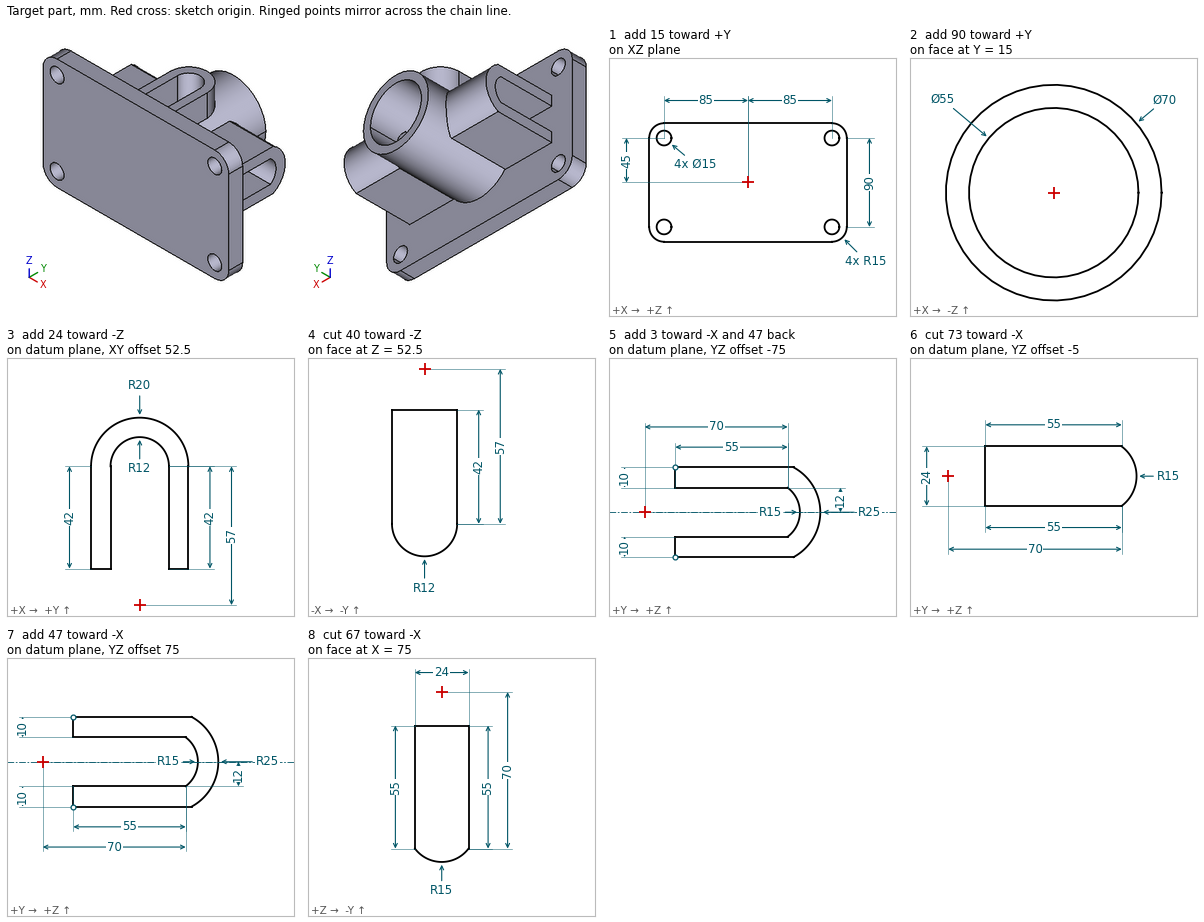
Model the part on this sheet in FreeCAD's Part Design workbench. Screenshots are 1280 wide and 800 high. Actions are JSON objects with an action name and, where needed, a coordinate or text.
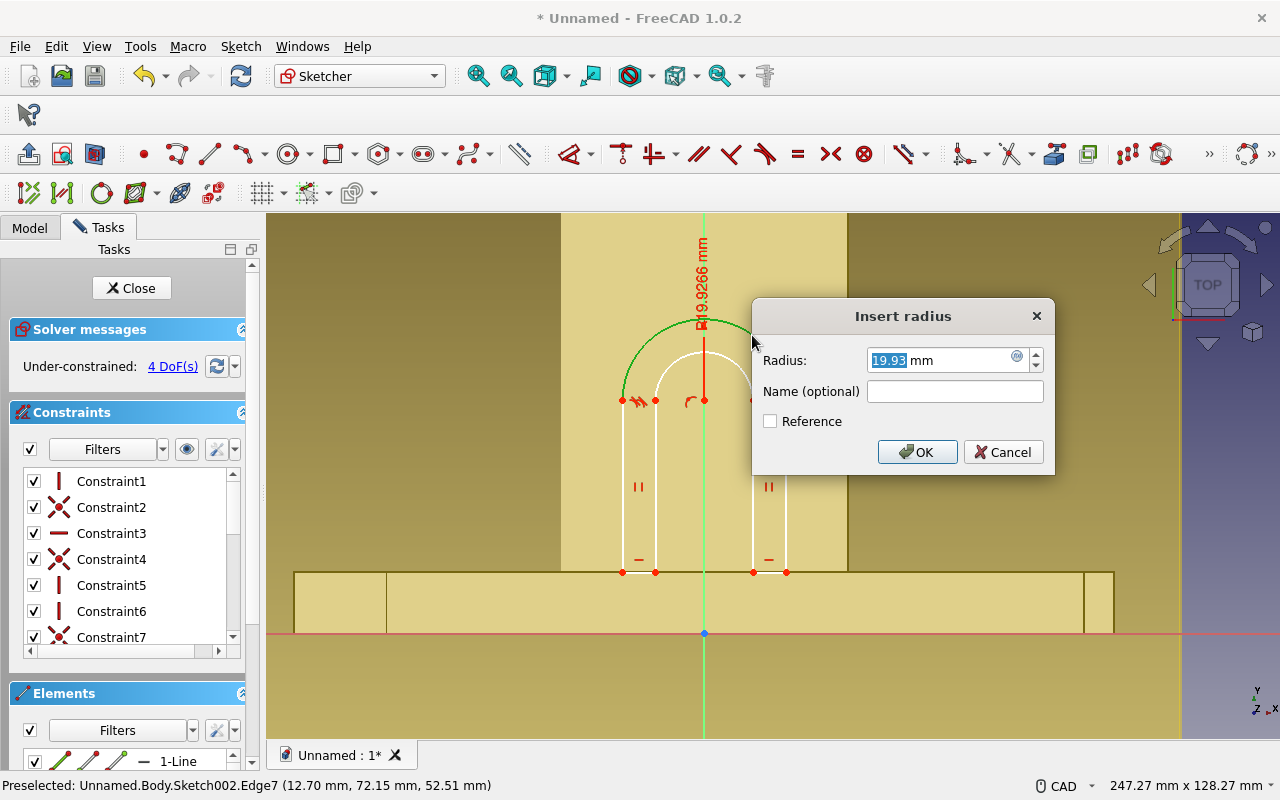
{"action": "type", "text": "20"}
{"action": "key", "text": "Return"}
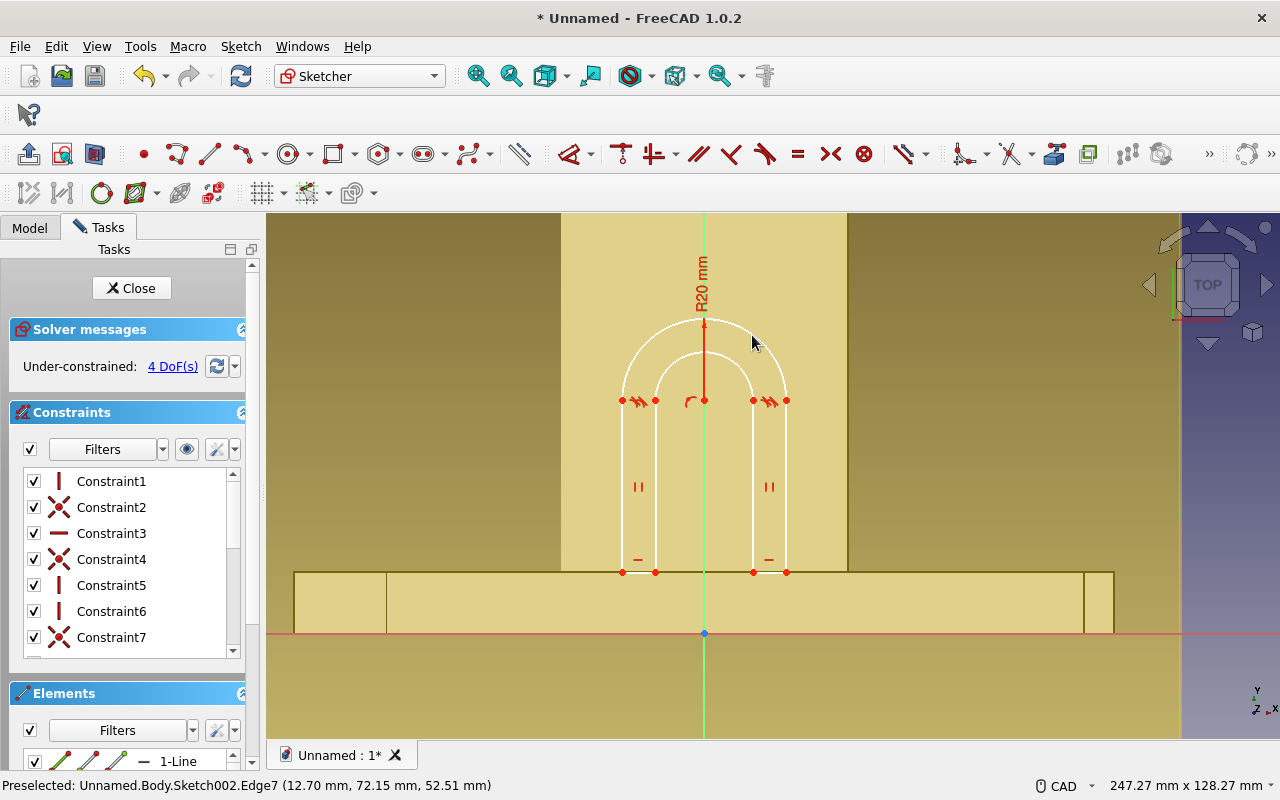
{"action": "left_click", "coordinate": [733, 362]}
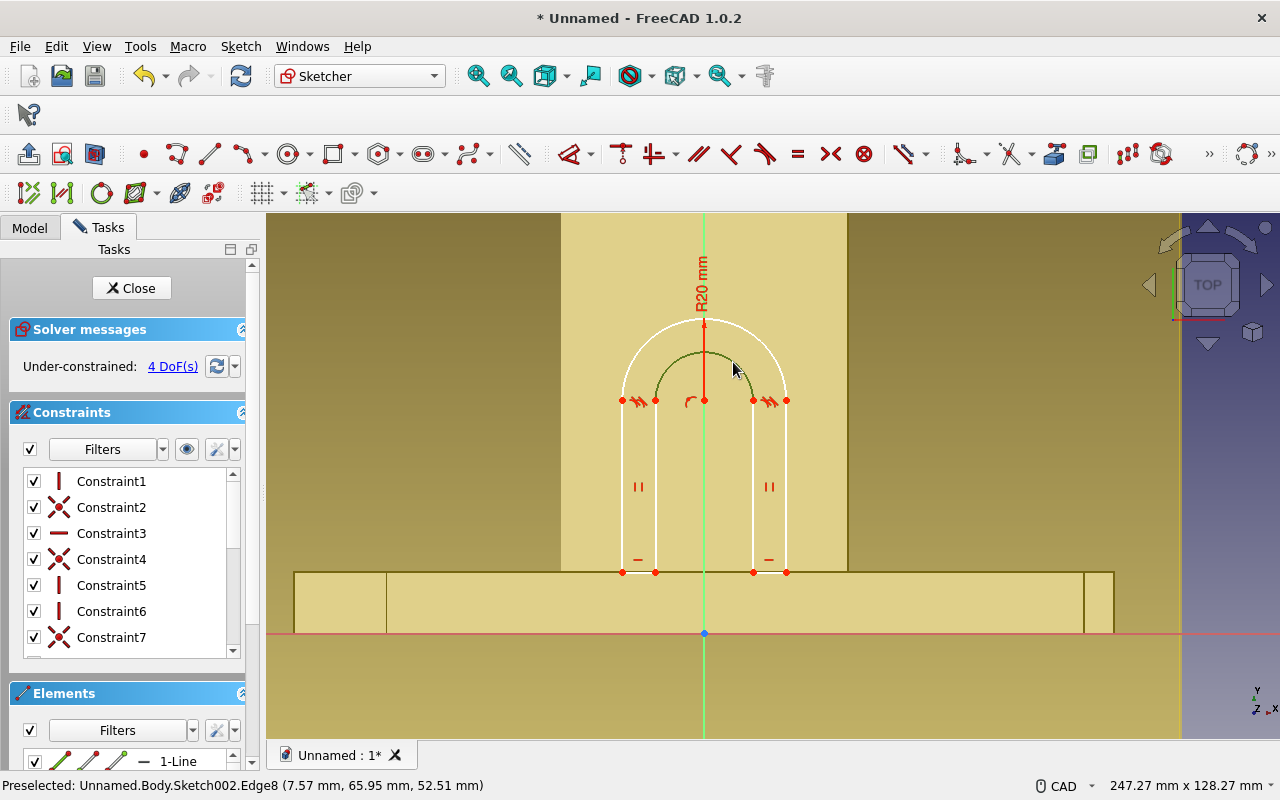
{"action": "key", "text": "k r"}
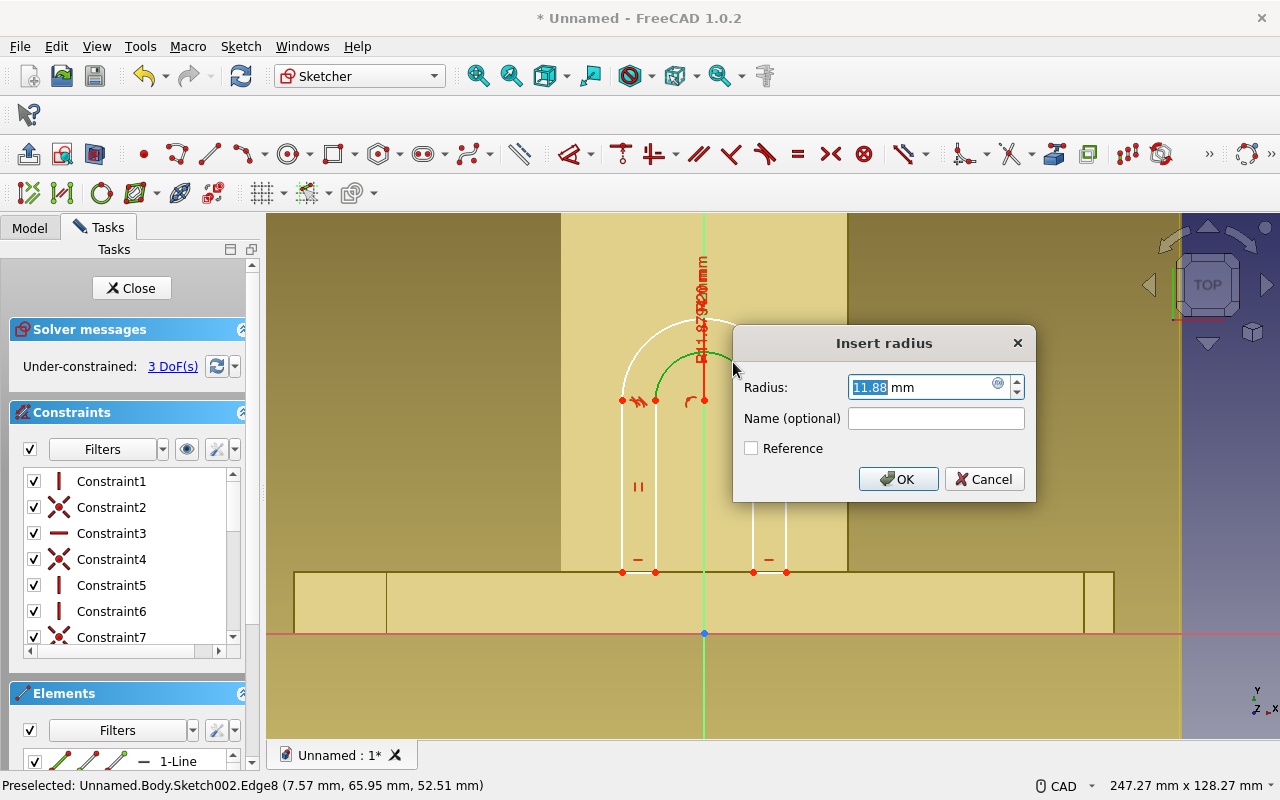
{"action": "type", "text": "12"}
{"action": "key", "text": "Return"}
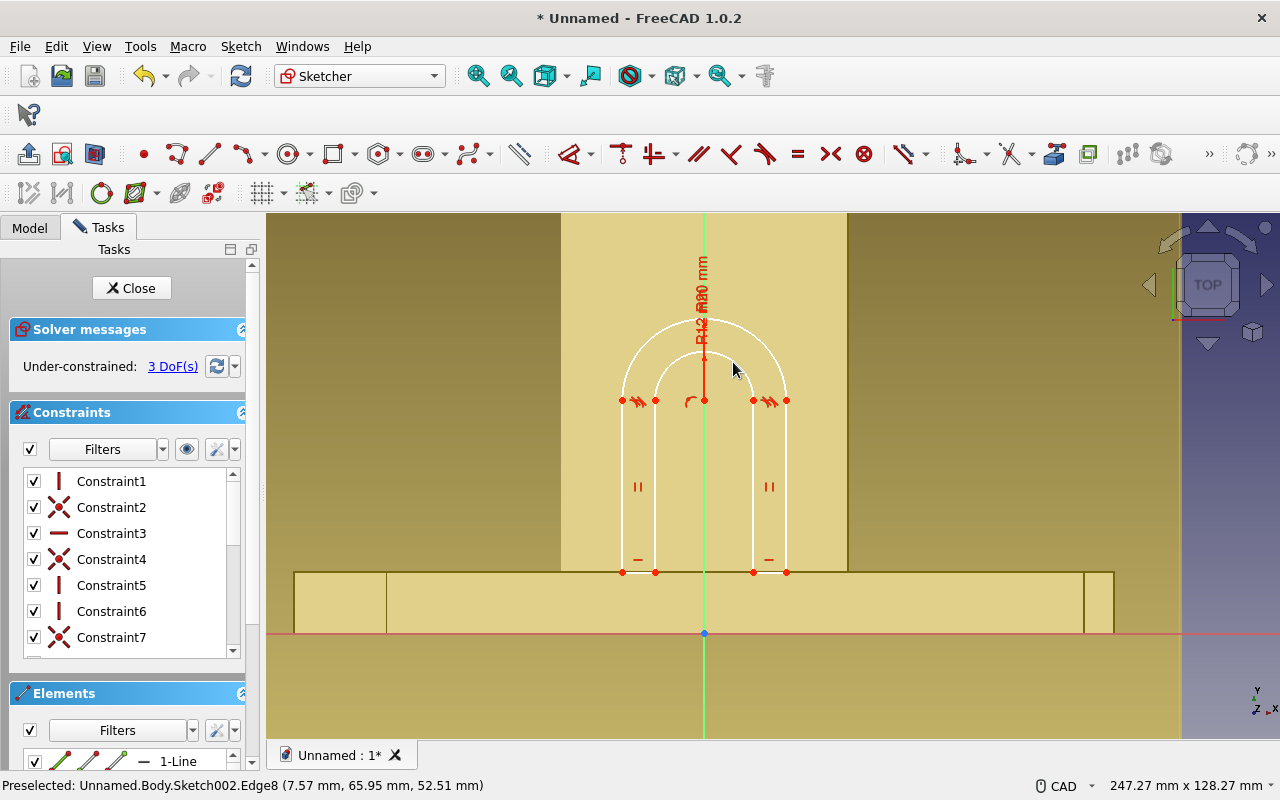
{"action": "left_click", "coordinate": [753, 453]}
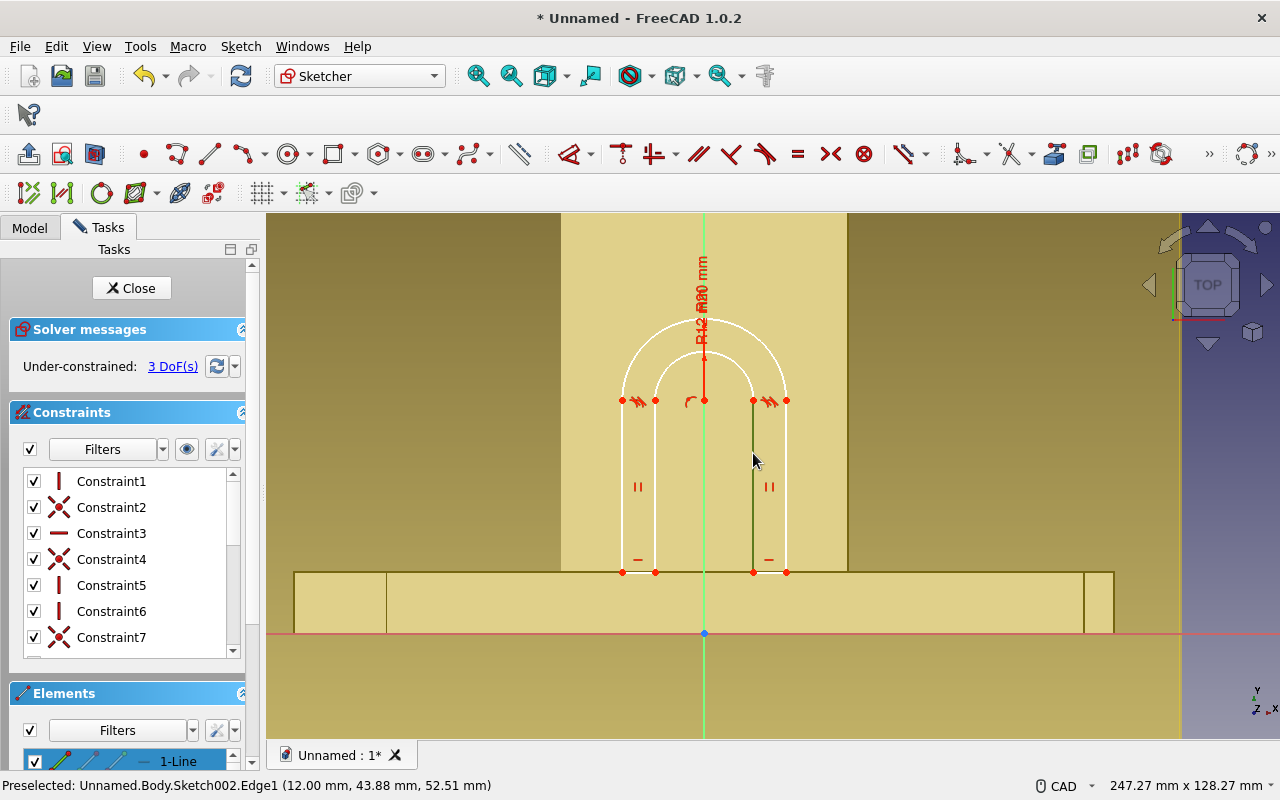
{"action": "key", "text": "i"}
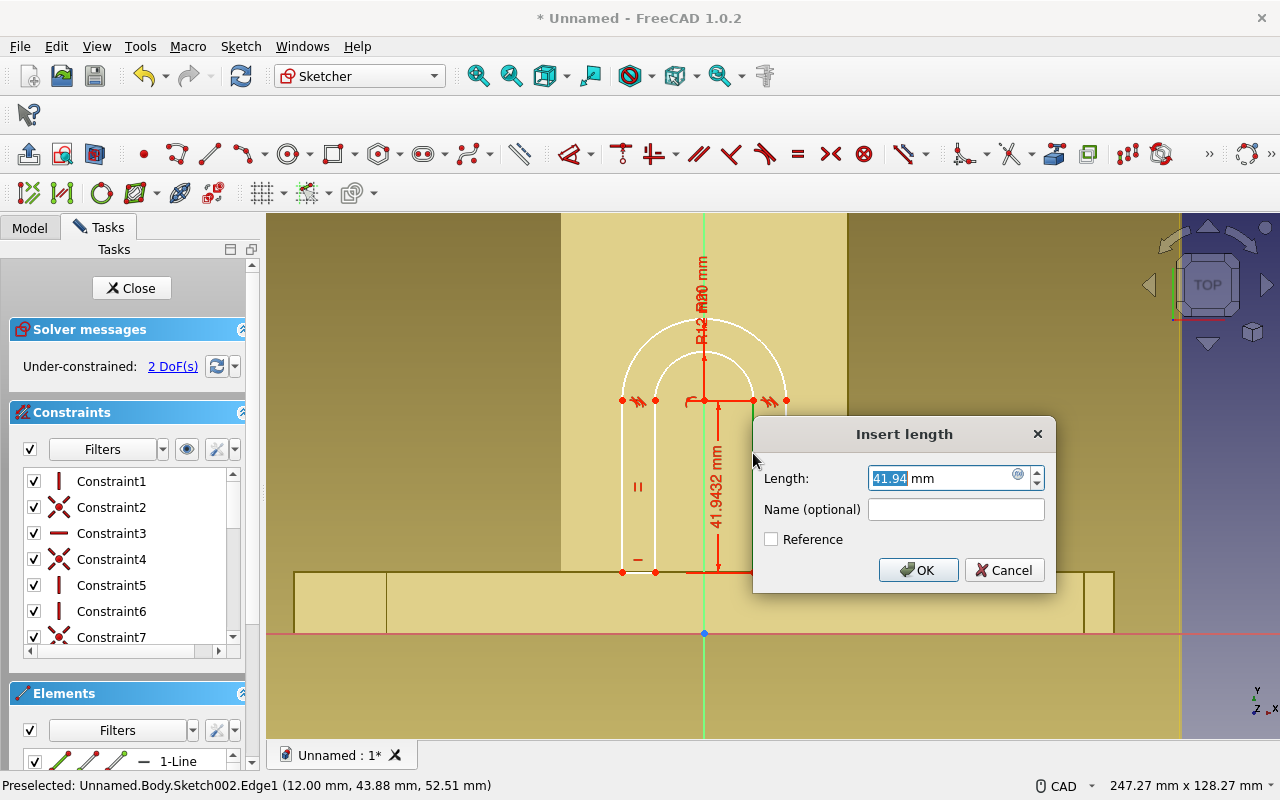
{"action": "type", "text": "42"}
{"action": "key", "text": "Return"}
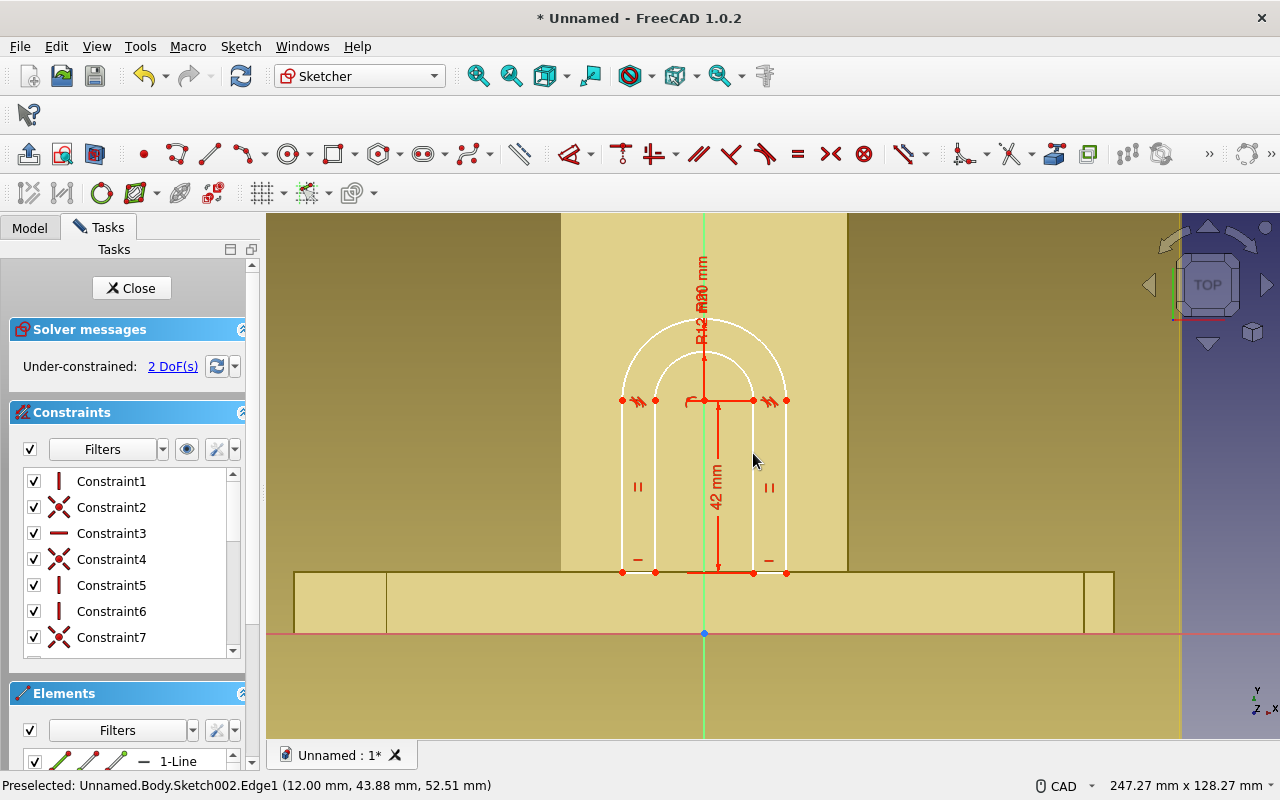
{"action": "left_click", "coordinate": [622, 453]}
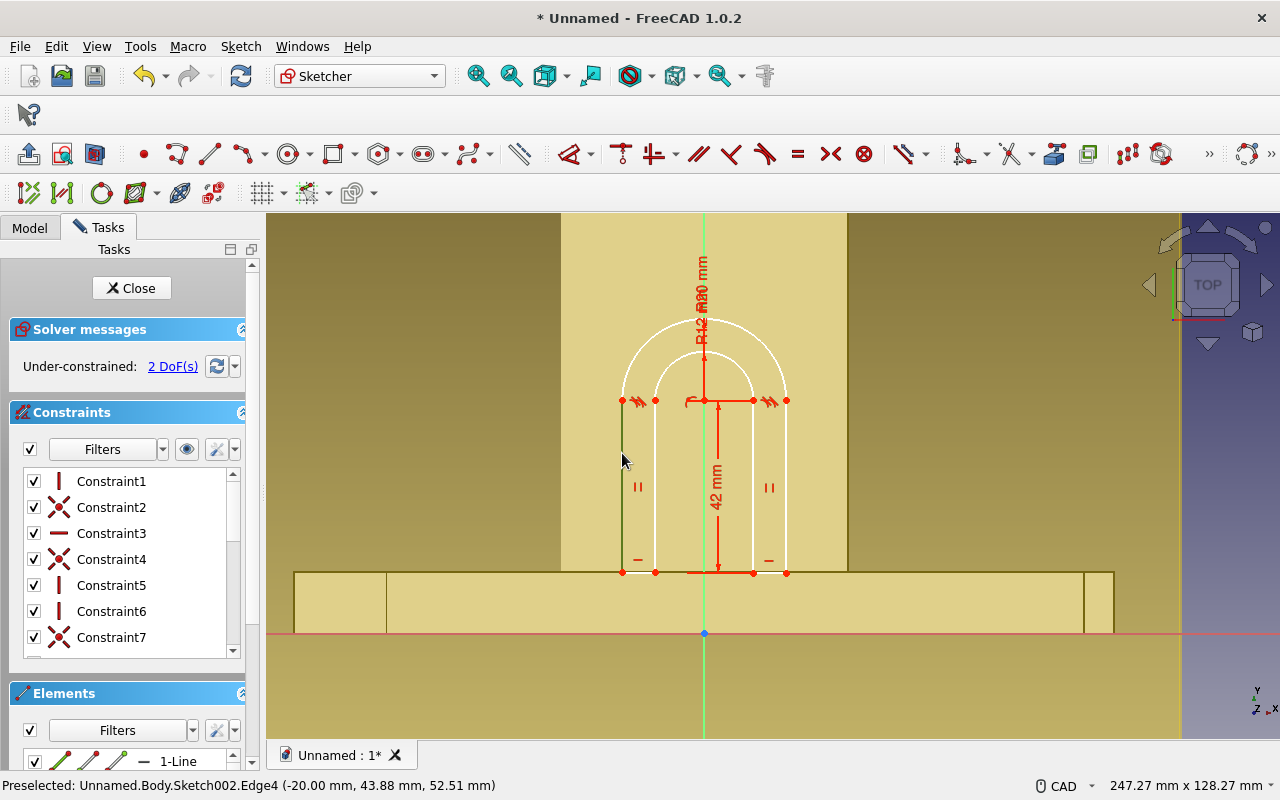
{"action": "key", "text": "i"}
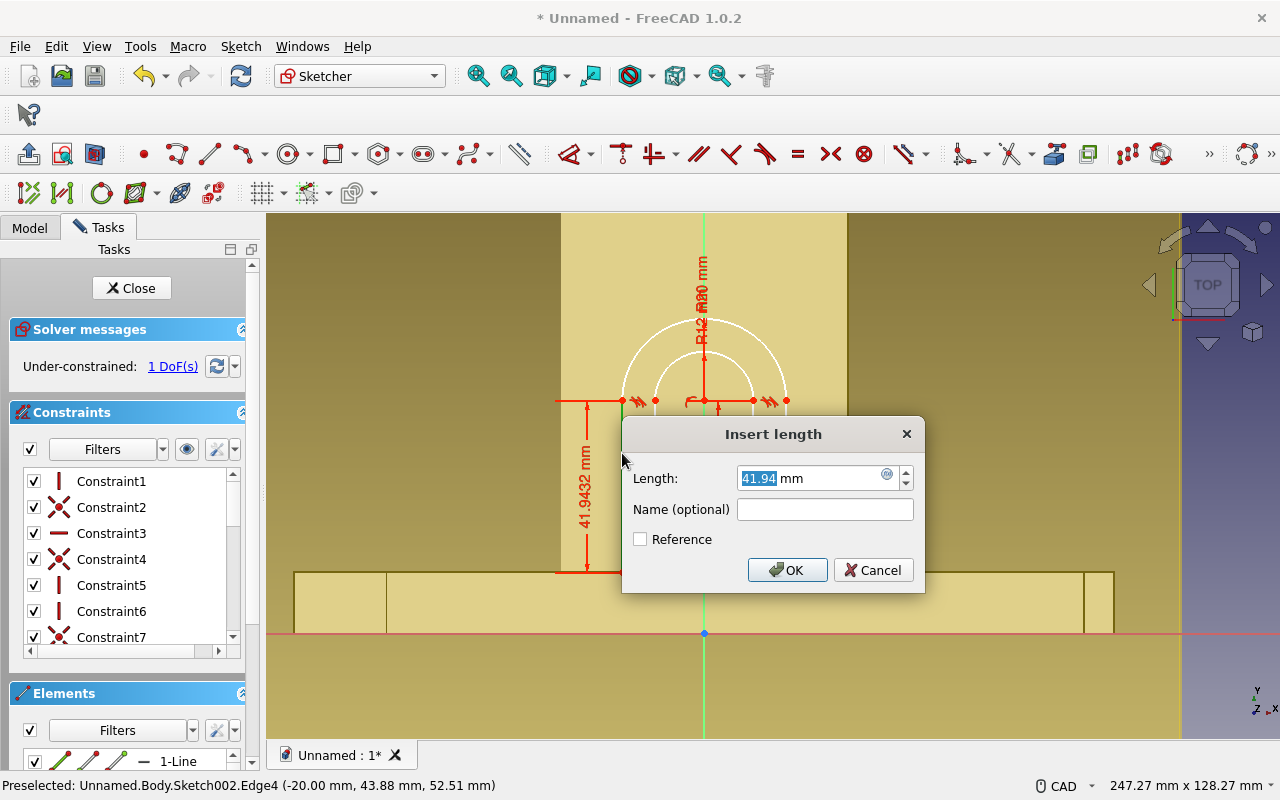
{"action": "type", "text": "42"}
{"action": "key", "text": "Return"}